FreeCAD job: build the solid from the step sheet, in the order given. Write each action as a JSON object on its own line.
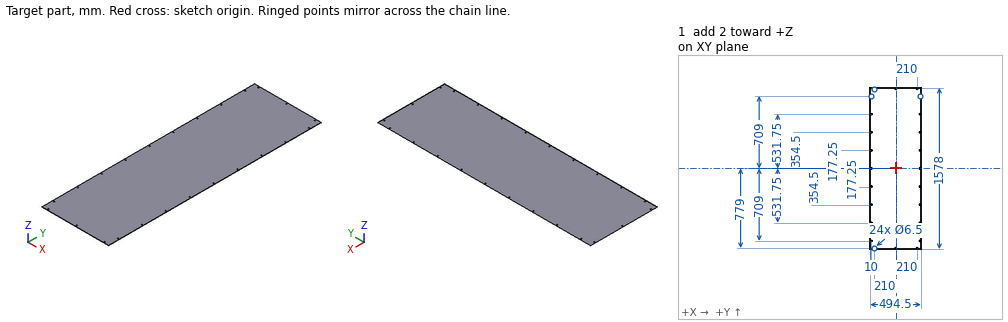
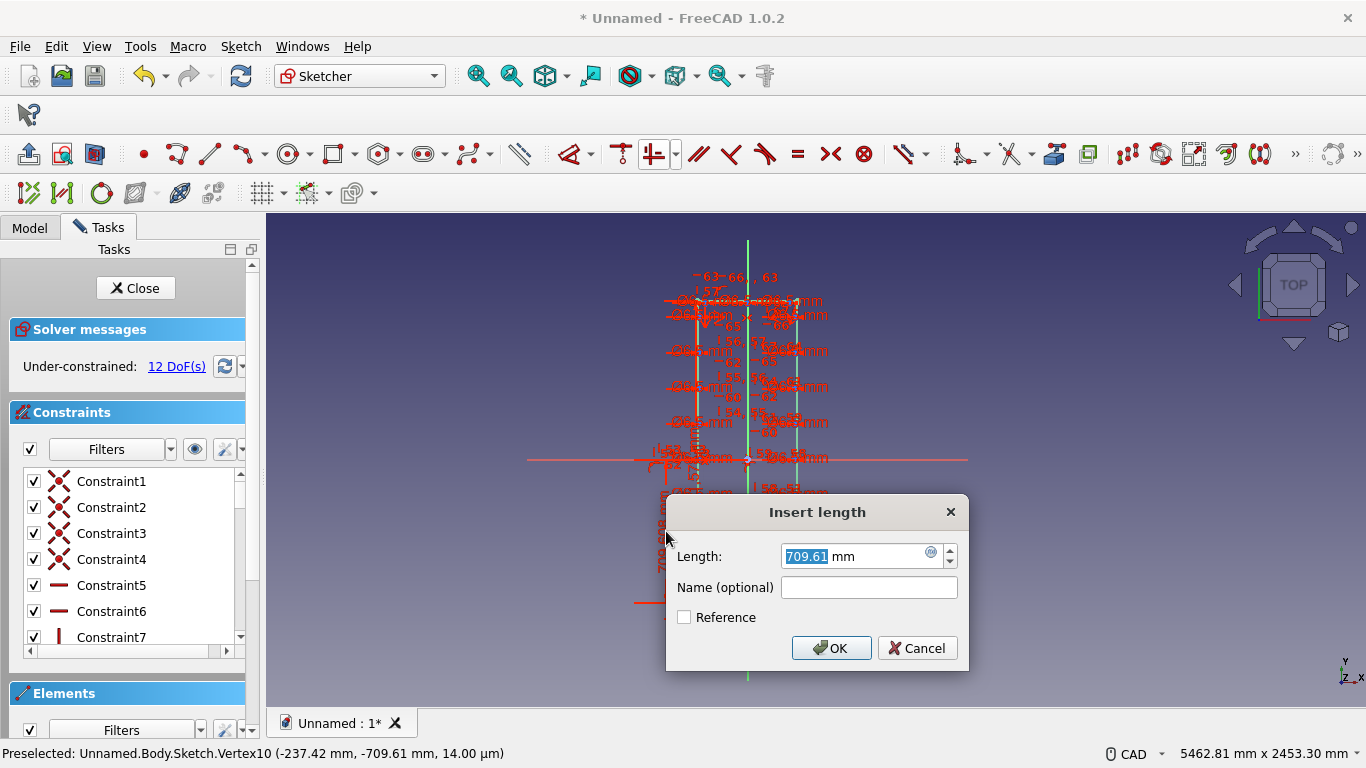
{"action": "type", "text": "709"}
{"action": "key", "text": "Return"}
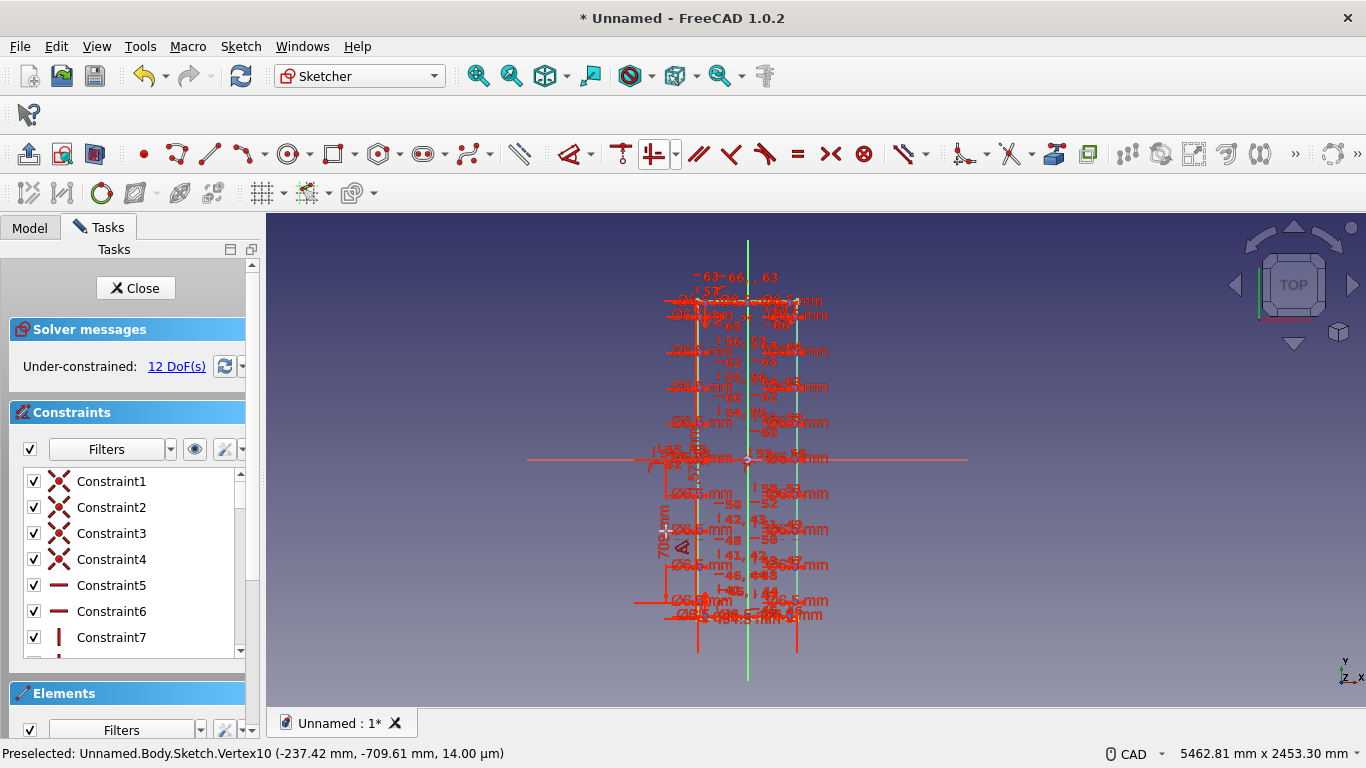
{"action": "scroll", "coordinate": [705, 617], "scroll_direction": "up", "scroll_amount": 3}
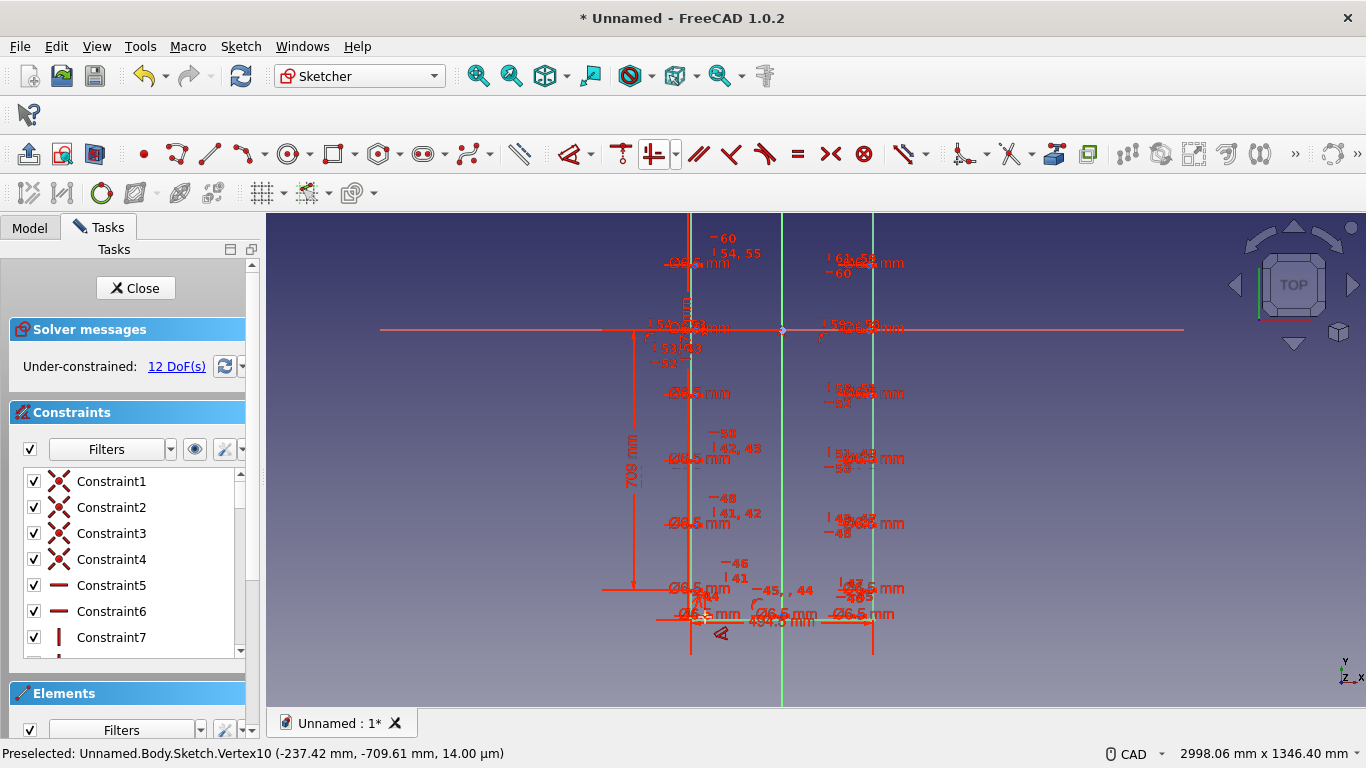
{"action": "left_click", "coordinate": [705, 616]}
{"action": "left_click", "coordinate": [744, 650]}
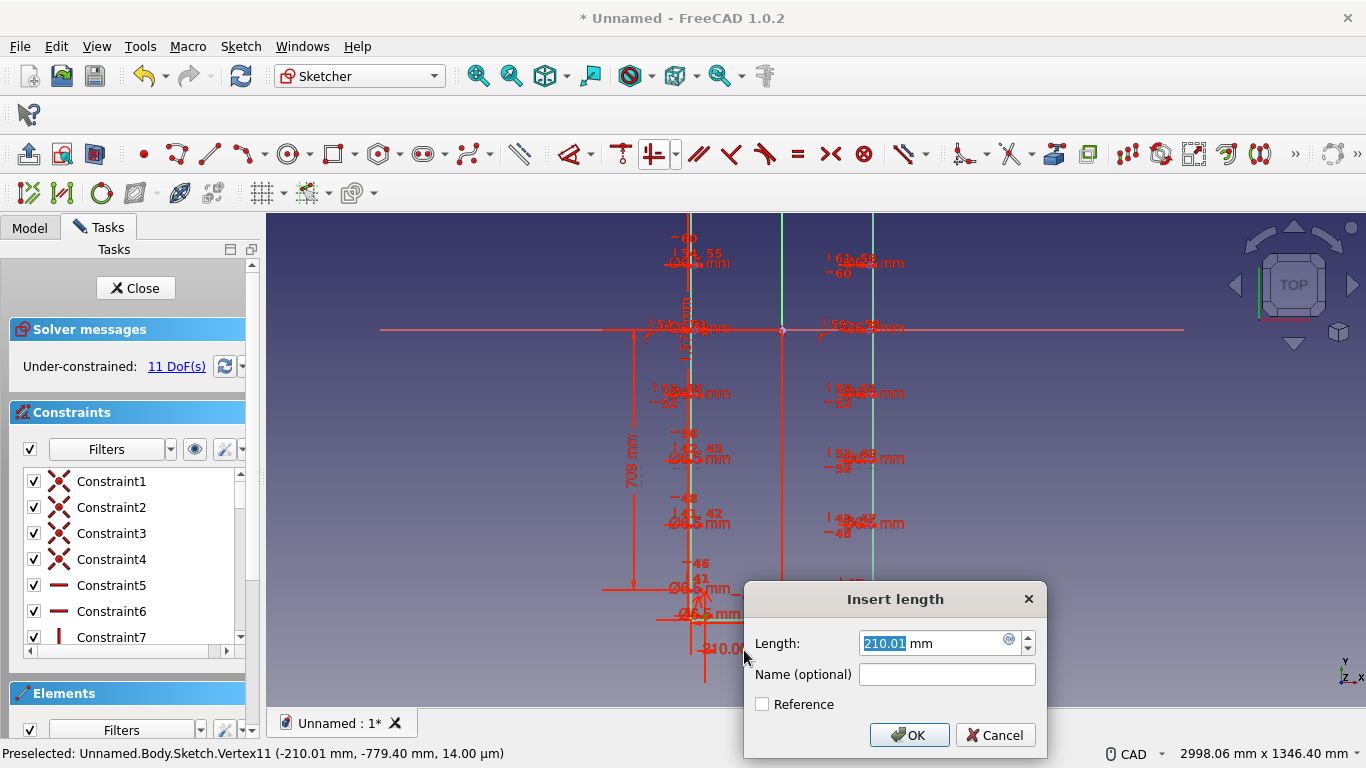
{"action": "type", "text": "210"}
{"action": "key", "text": "Return"}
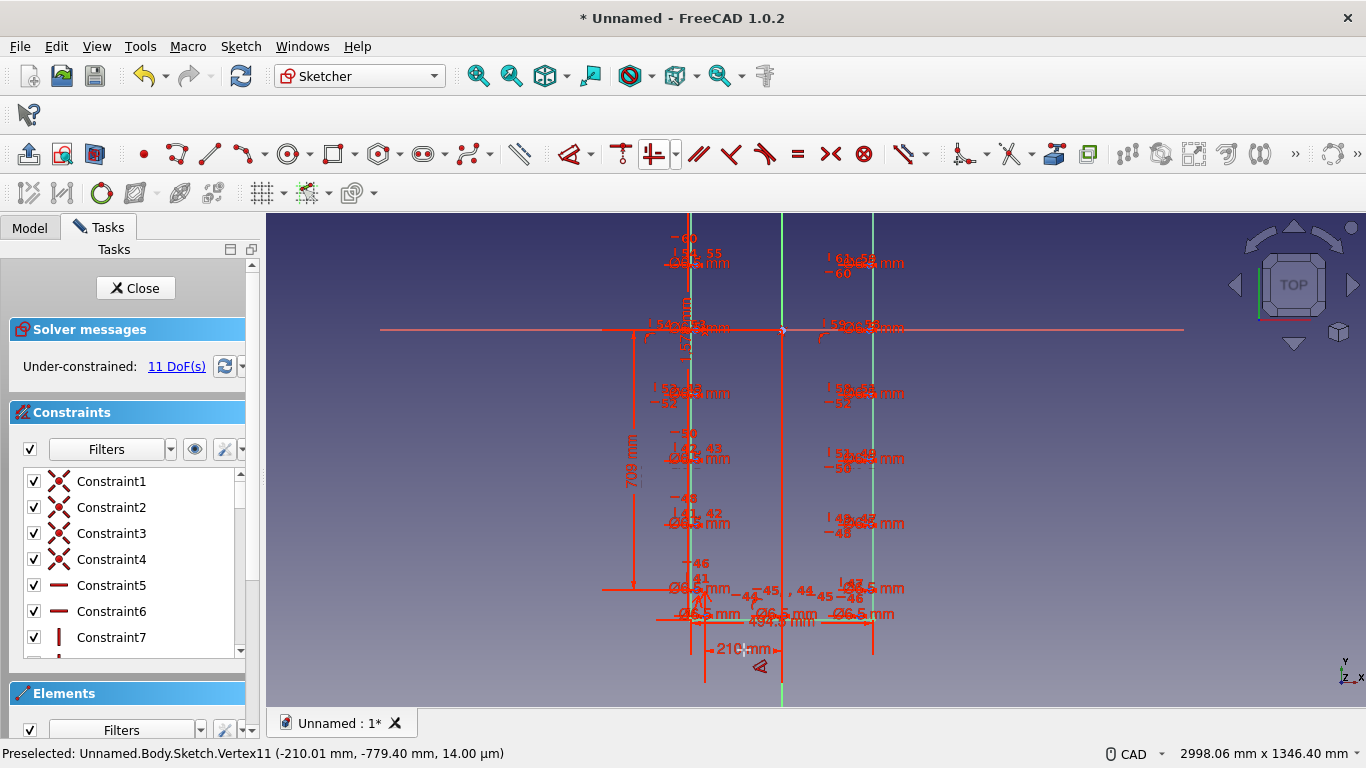
{"action": "left_click", "coordinate": [705, 616]}
{"action": "left_click", "coordinate": [671, 407]}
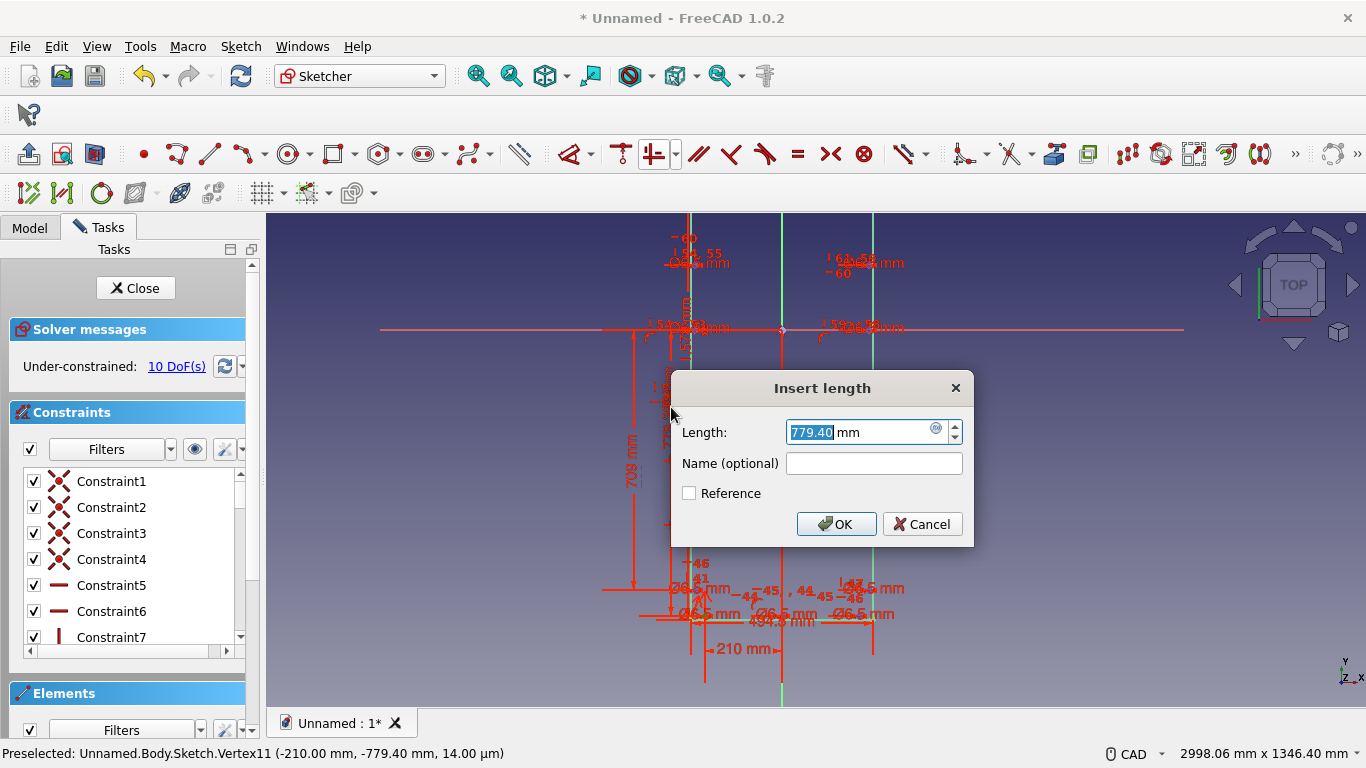
{"action": "type", "text": "779"}
{"action": "key", "text": "Return"}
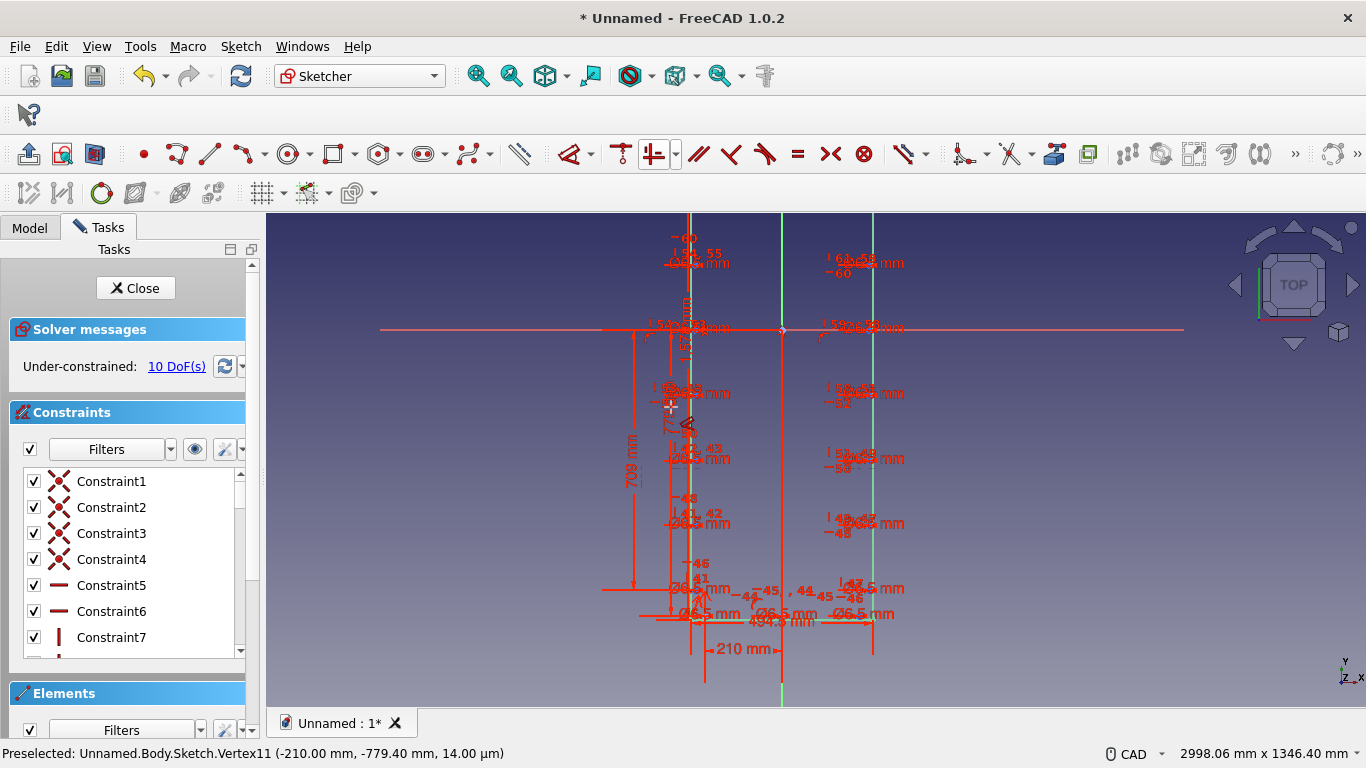
{"action": "left_click", "coordinate": [859, 616]}
{"action": "left_click", "coordinate": [821, 650]}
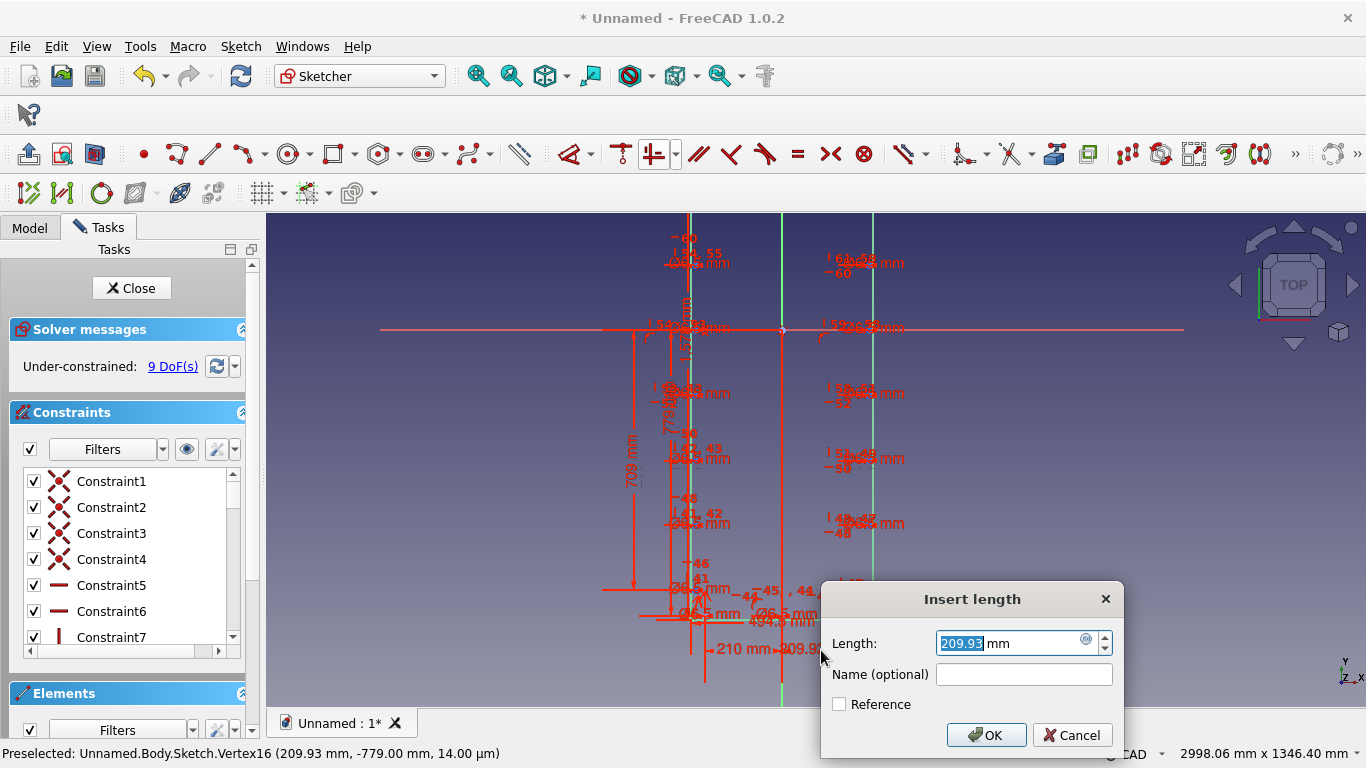
{"action": "type", "text": "210"}
{"action": "key", "text": "Return"}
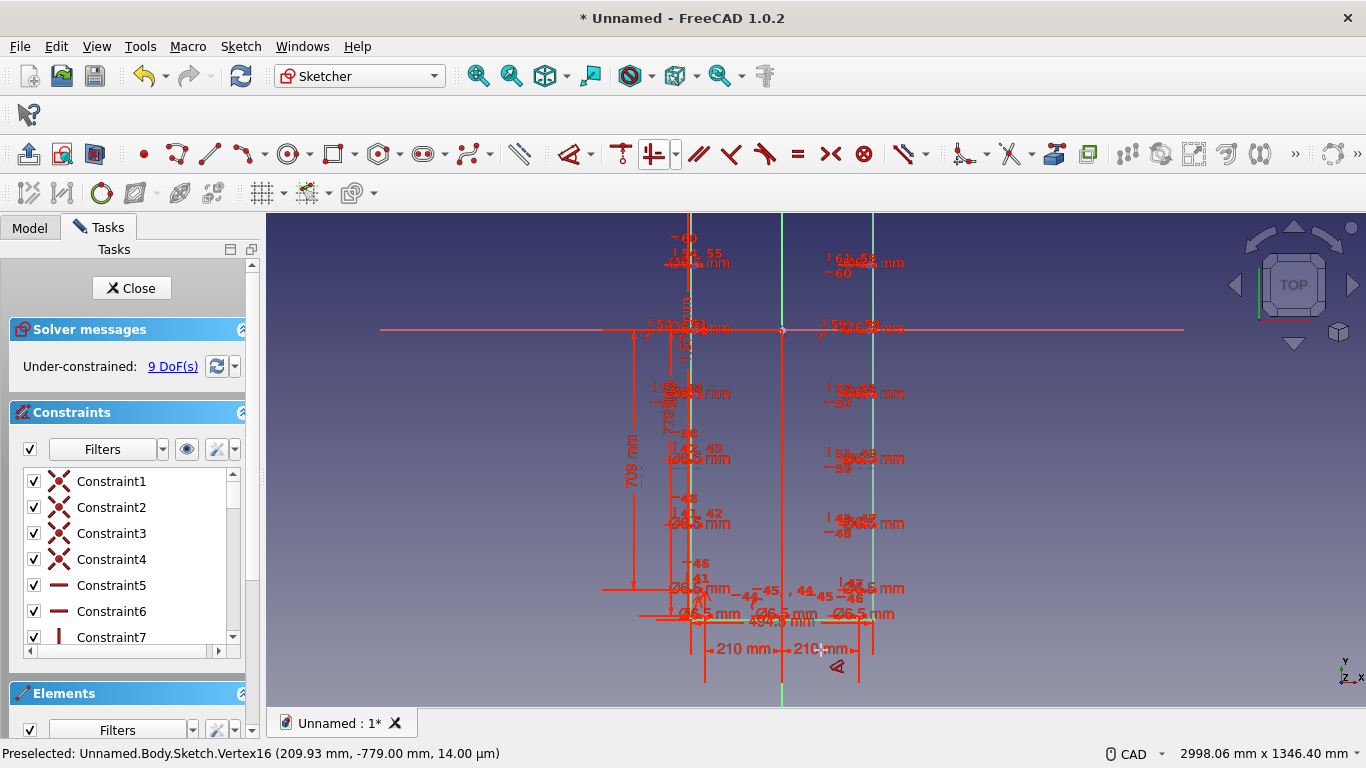
{"action": "scroll", "coordinate": [705, 618], "scroll_direction": "down", "scroll_amount": 3}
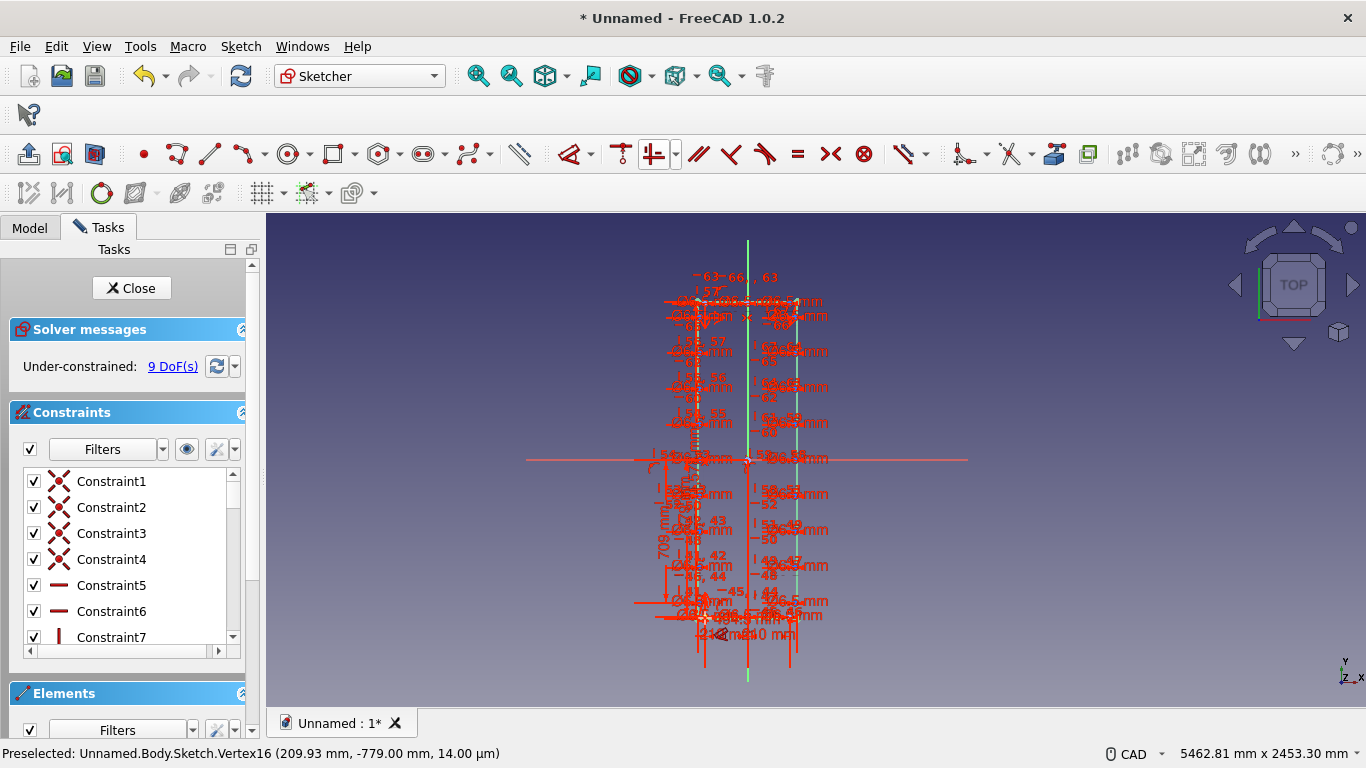
{"action": "left_click", "coordinate": [700, 318]}
{"action": "left_click", "coordinate": [666, 389]}